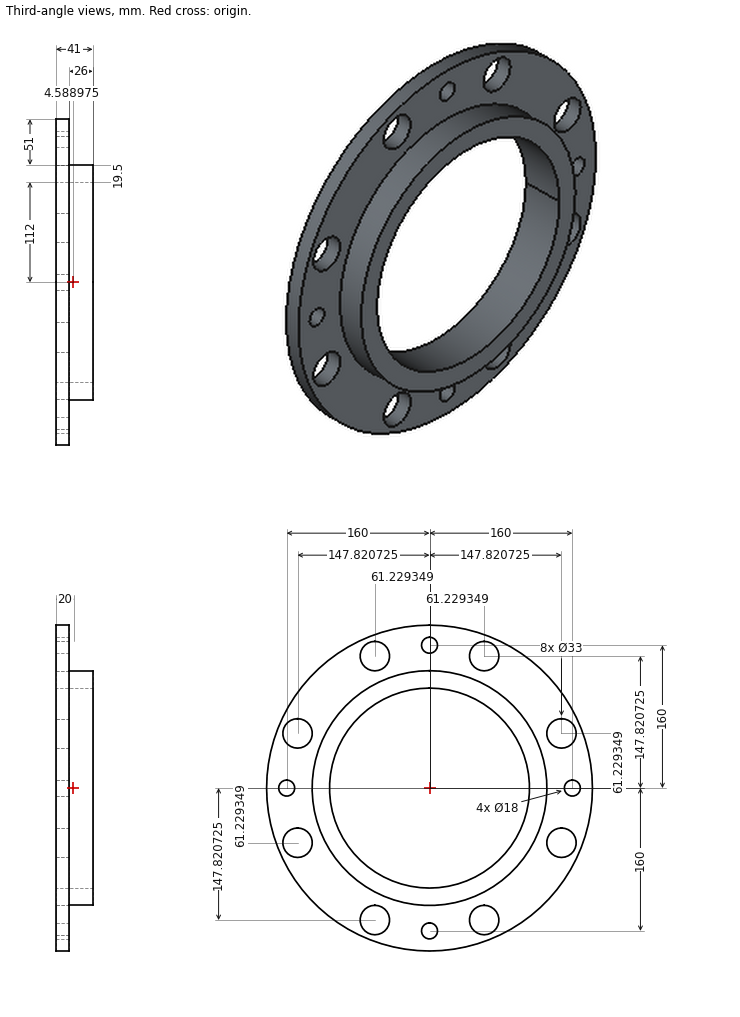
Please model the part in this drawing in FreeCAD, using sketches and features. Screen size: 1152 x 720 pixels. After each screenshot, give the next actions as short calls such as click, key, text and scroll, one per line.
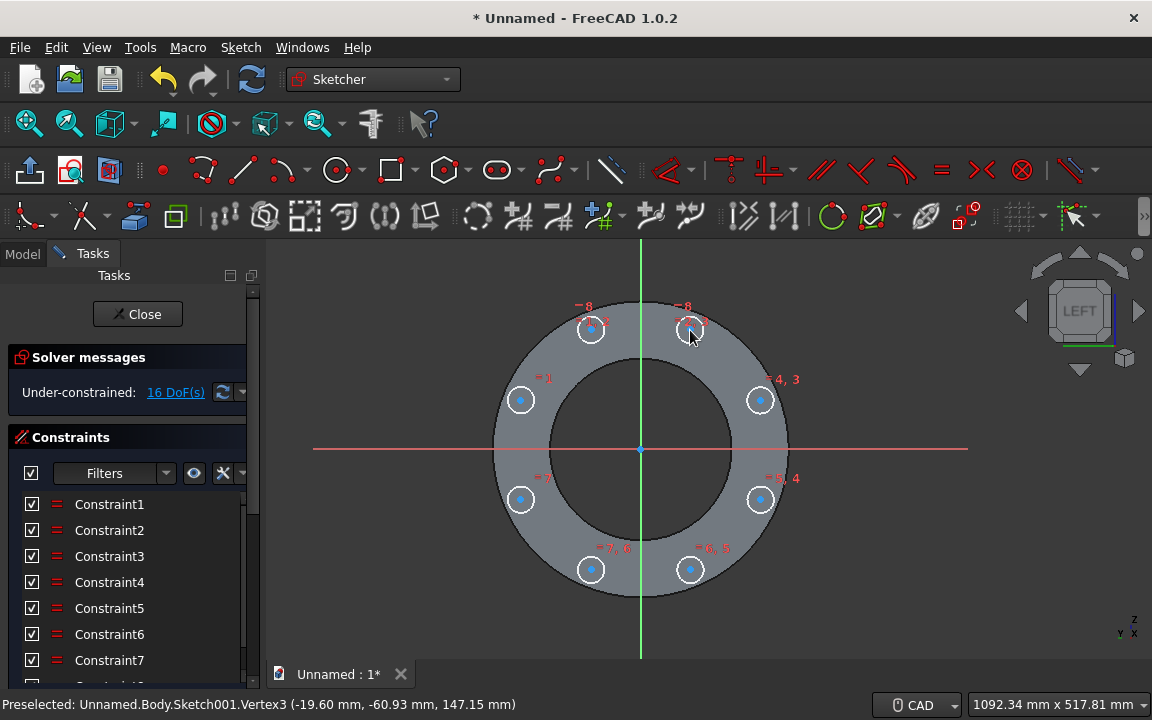
click(521, 400)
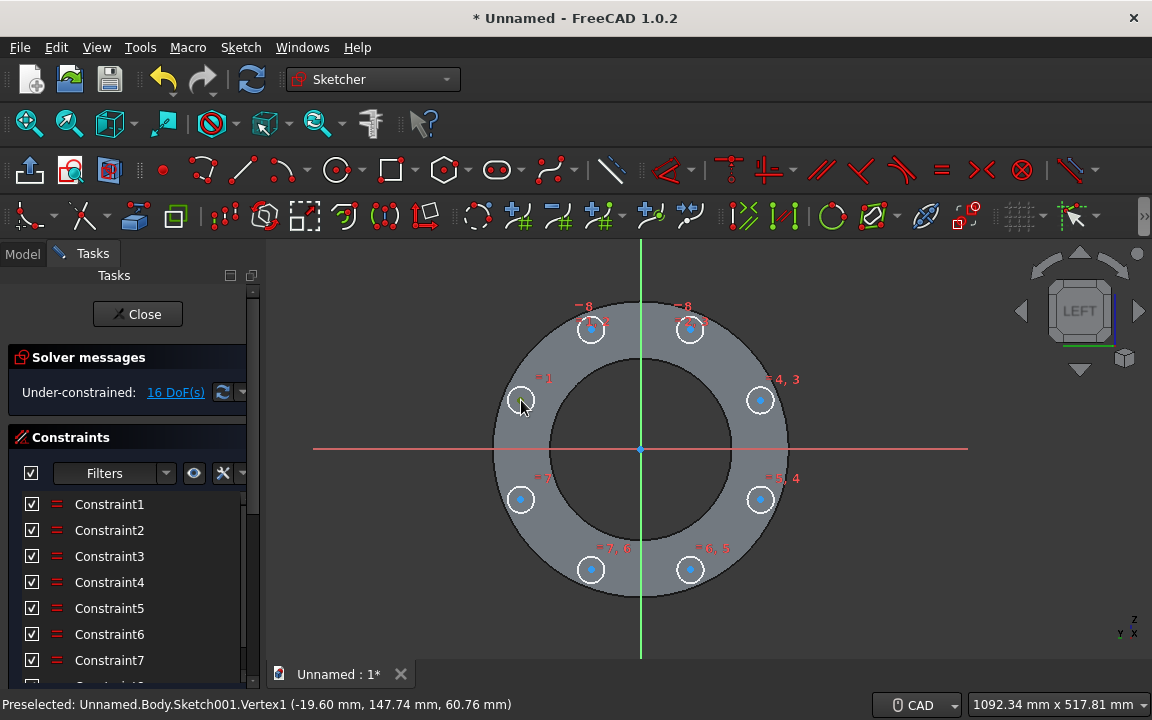
click(760, 400)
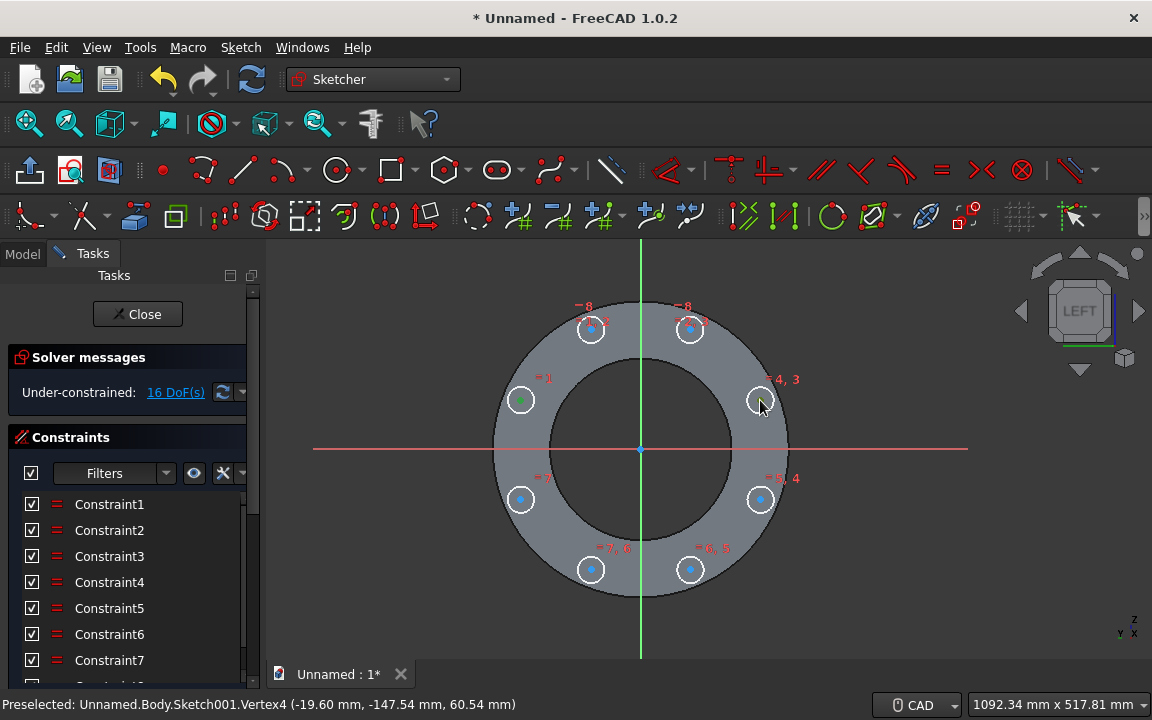
click(796, 170)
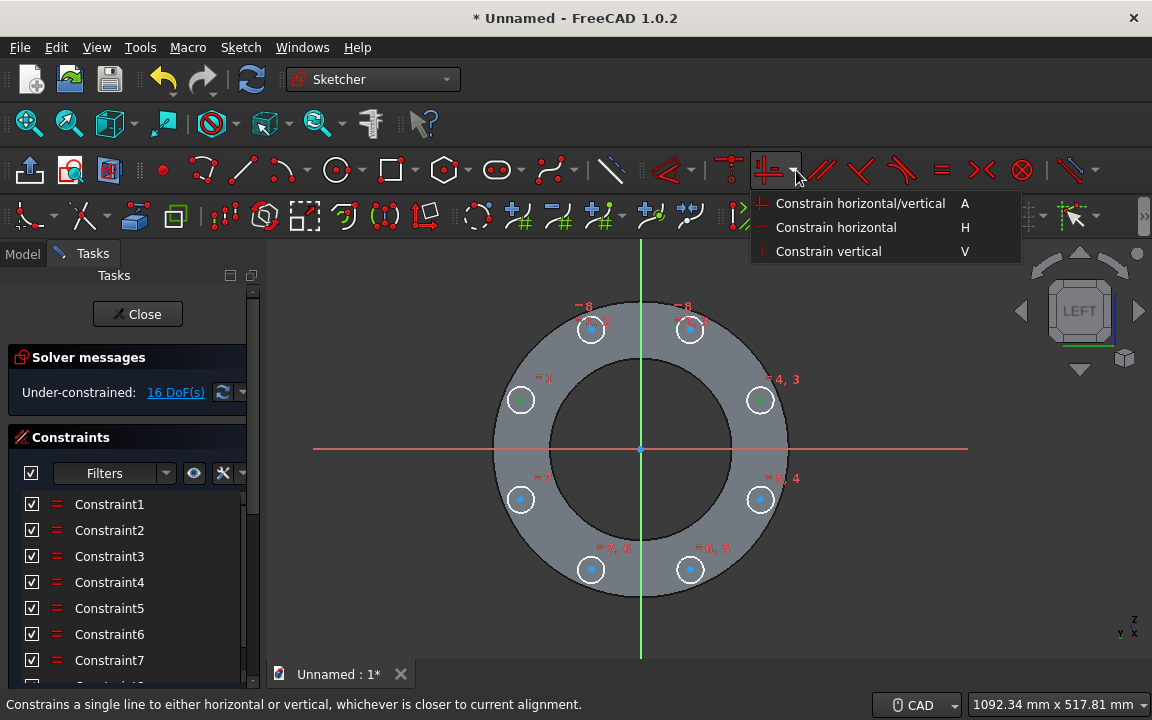
click(886, 227)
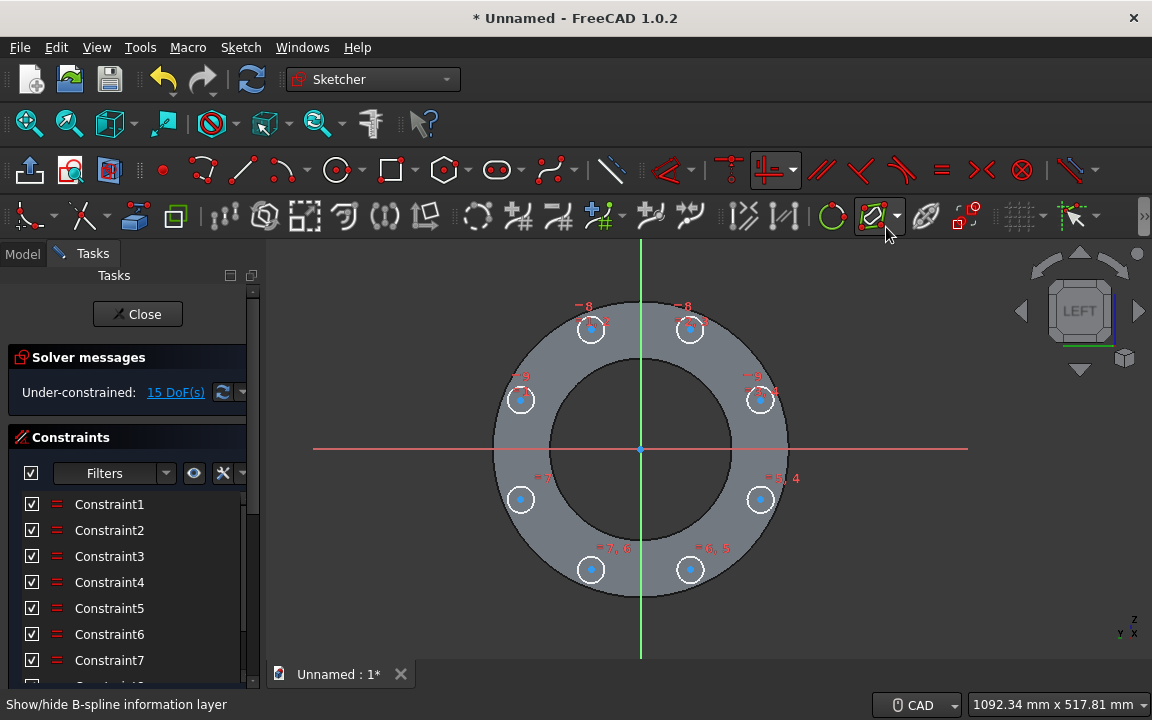
click(760, 400)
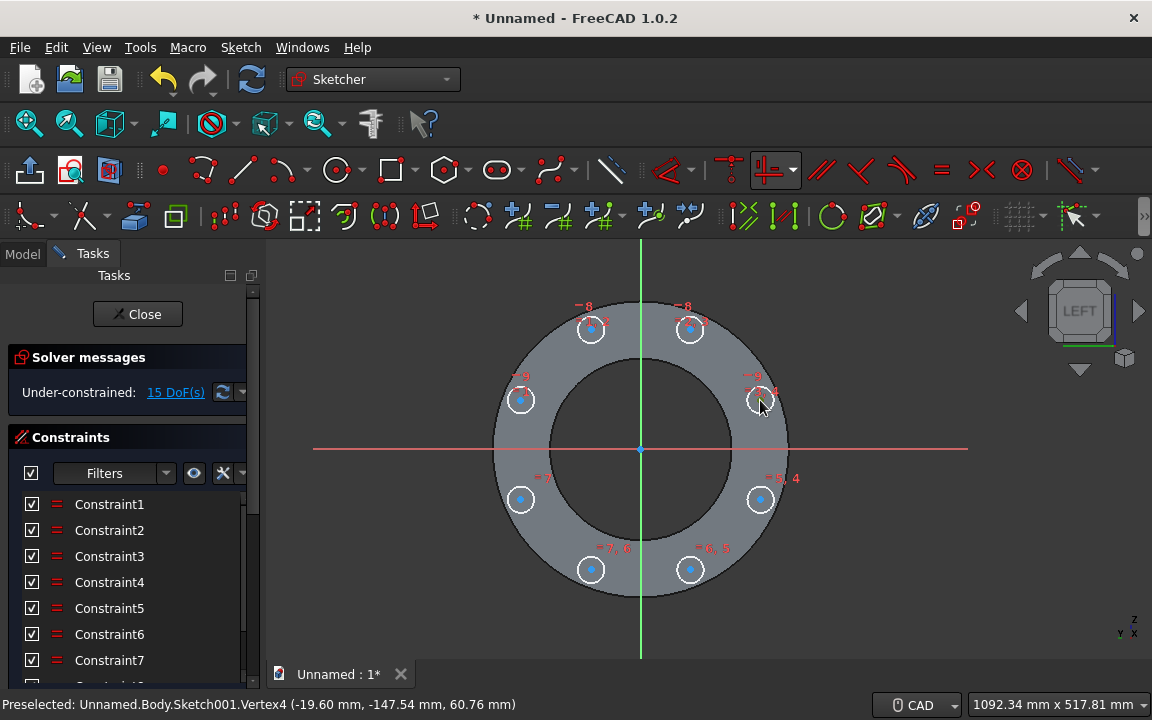
click(761, 500)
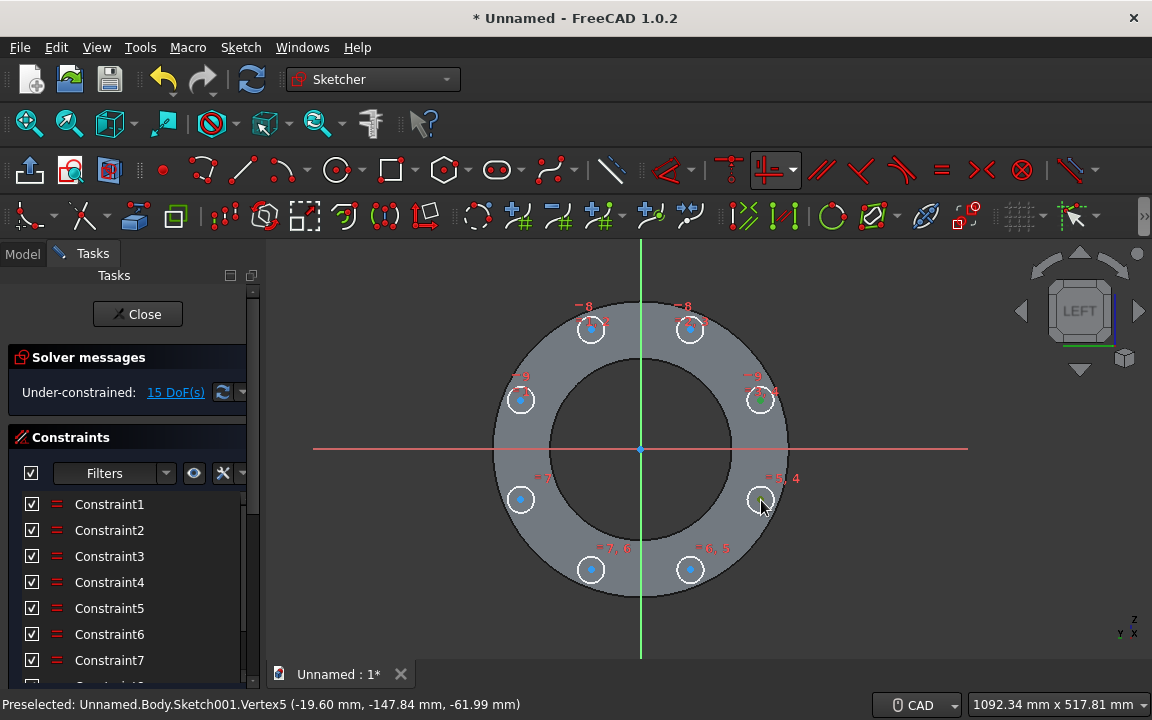
click(796, 170)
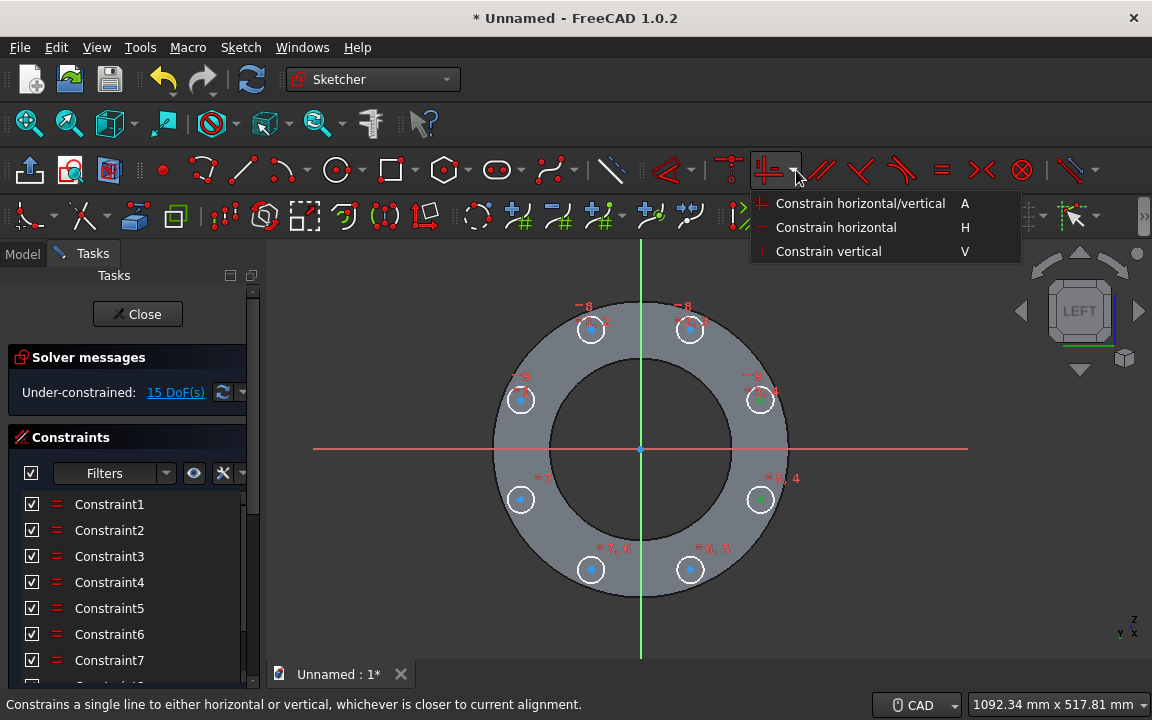
click(886, 251)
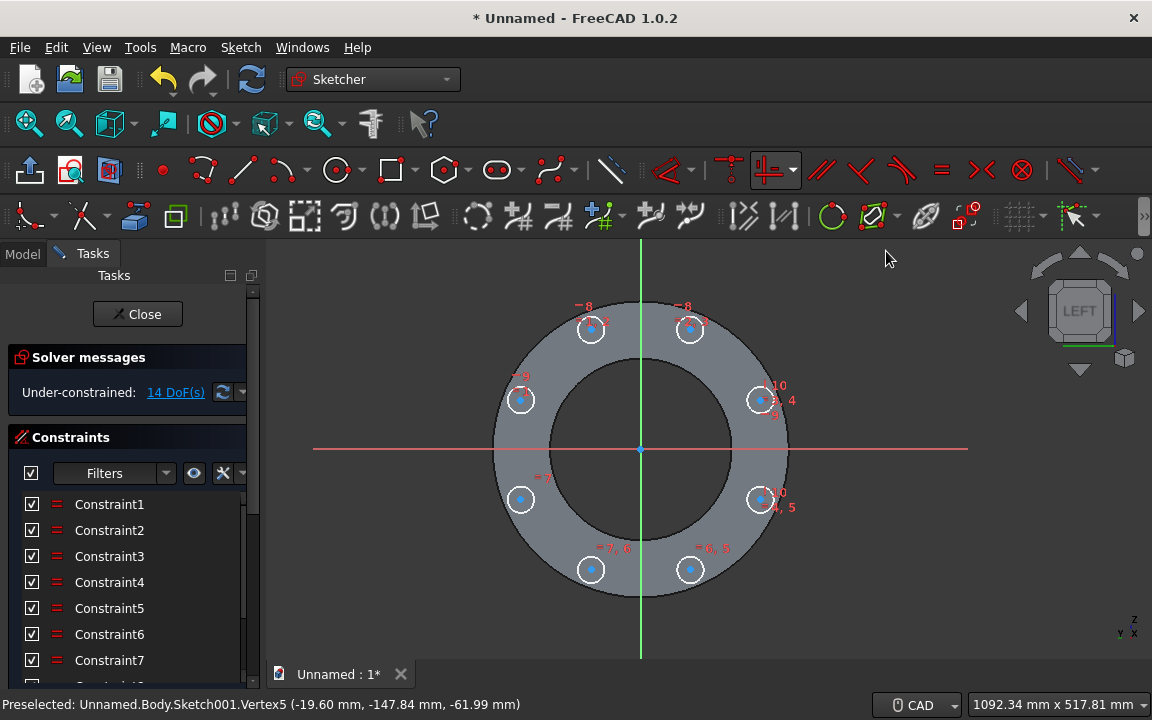
click(690, 330)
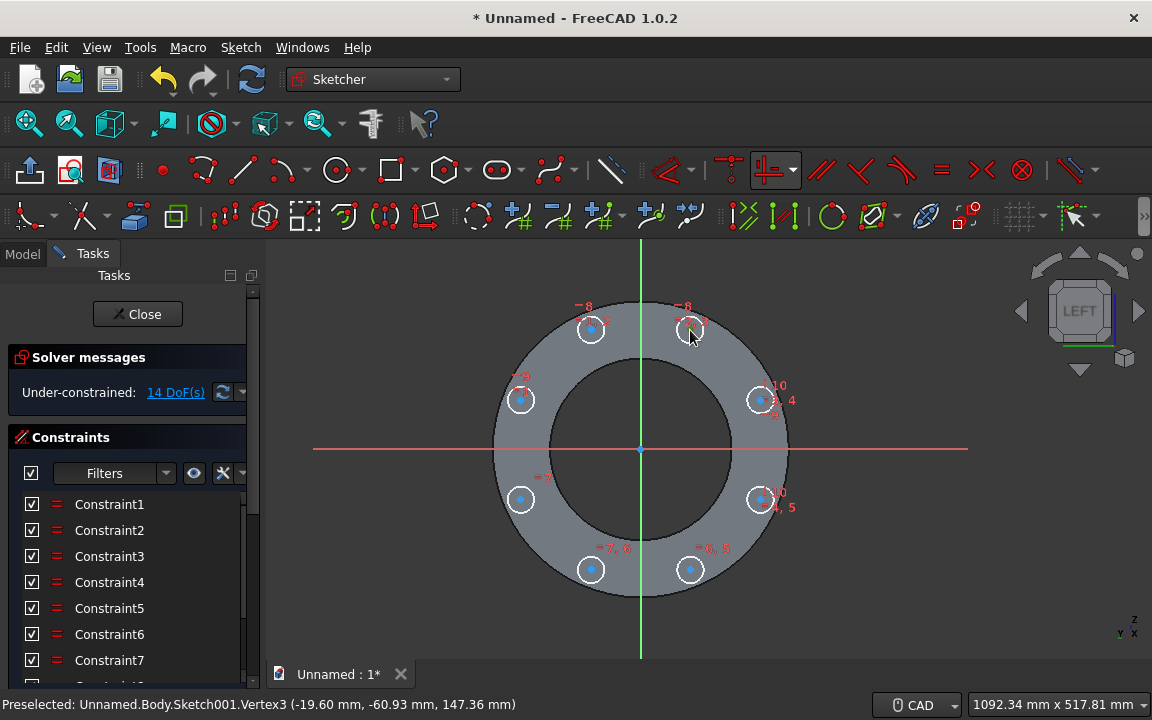
click(690, 570)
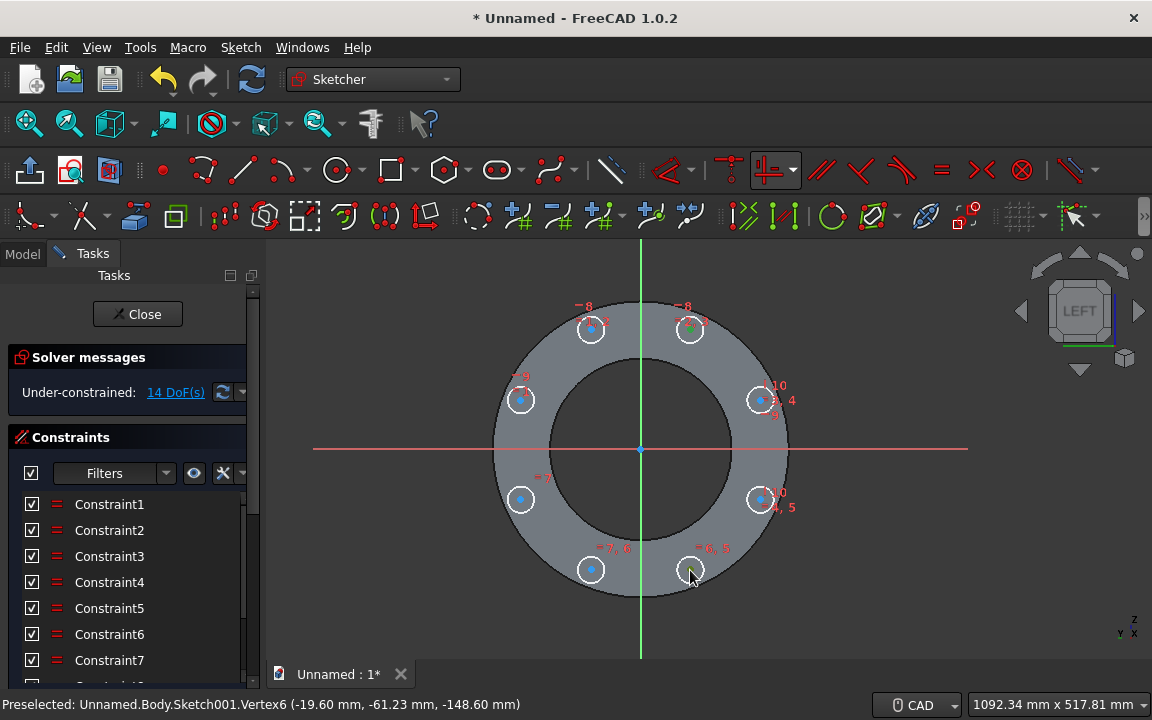
key(v)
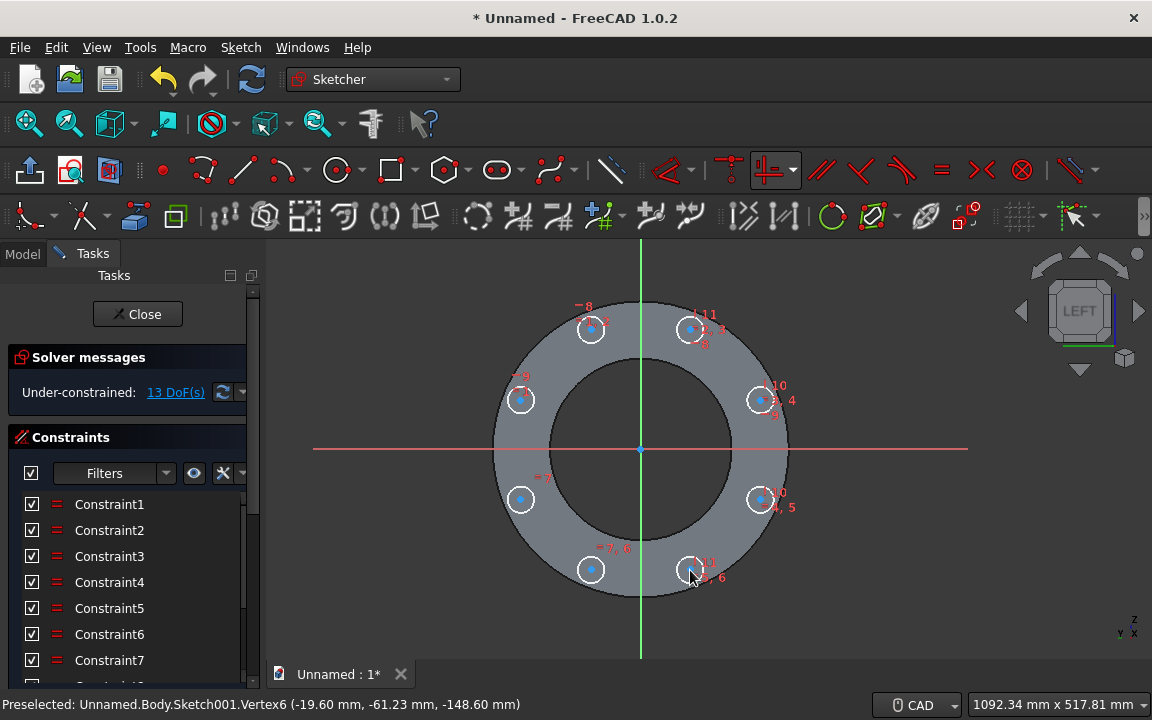
click(591, 330)